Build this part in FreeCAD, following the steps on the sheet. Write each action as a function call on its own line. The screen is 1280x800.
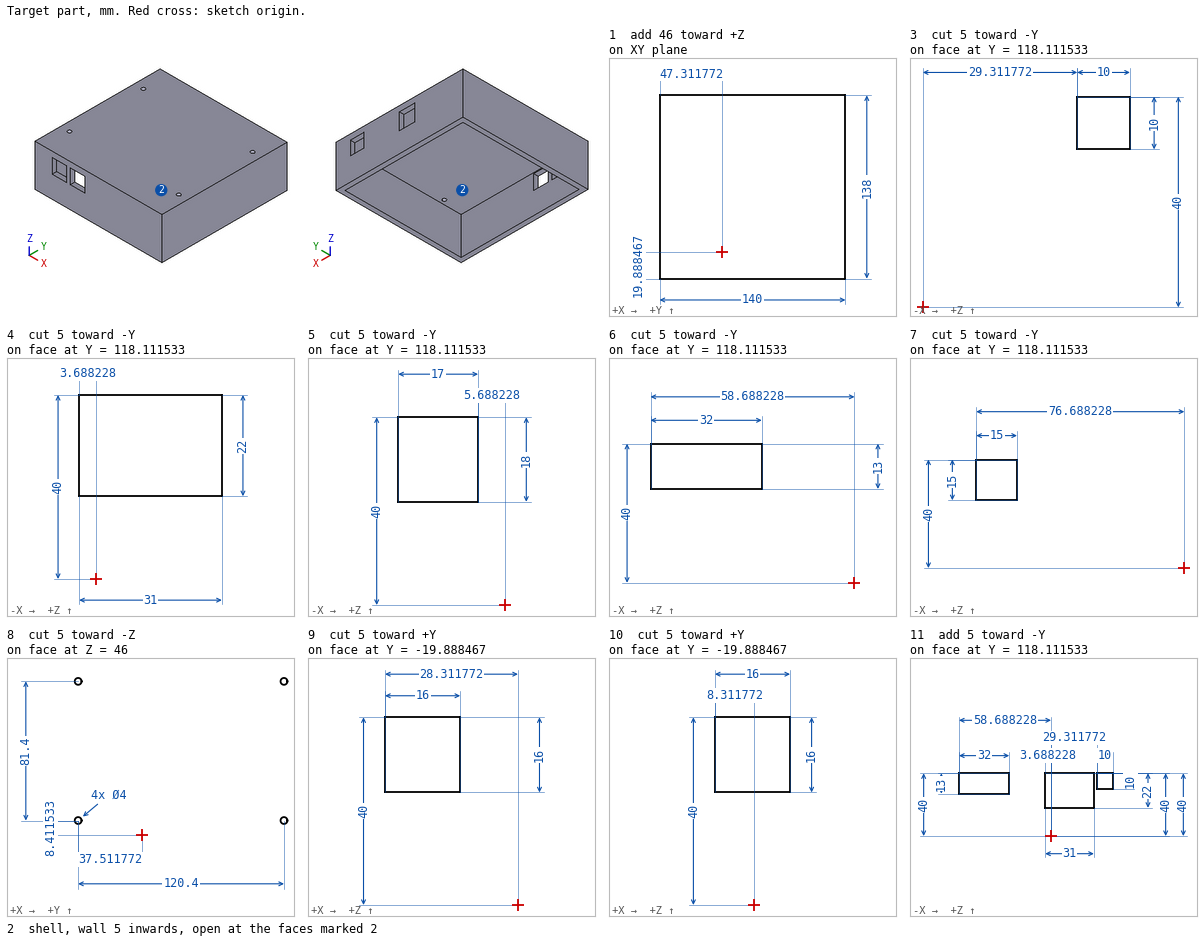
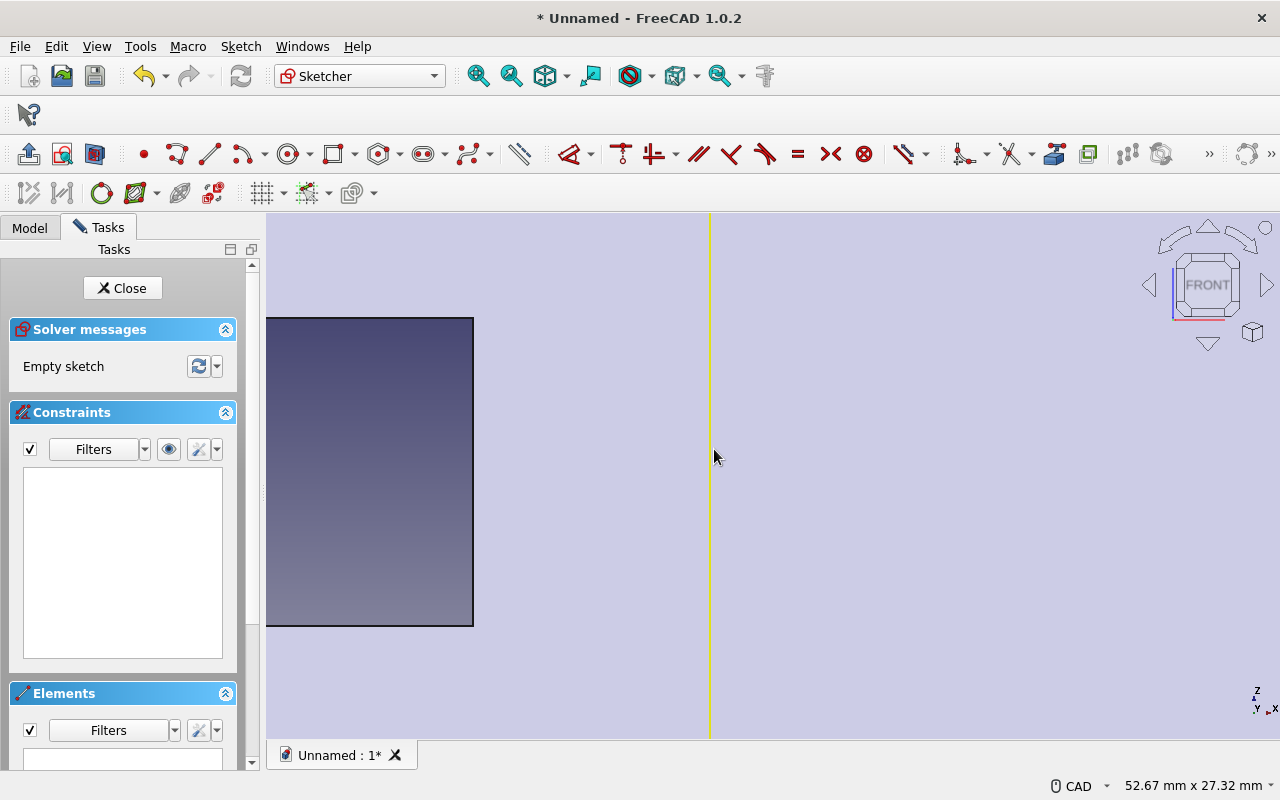
key(g)
key(r)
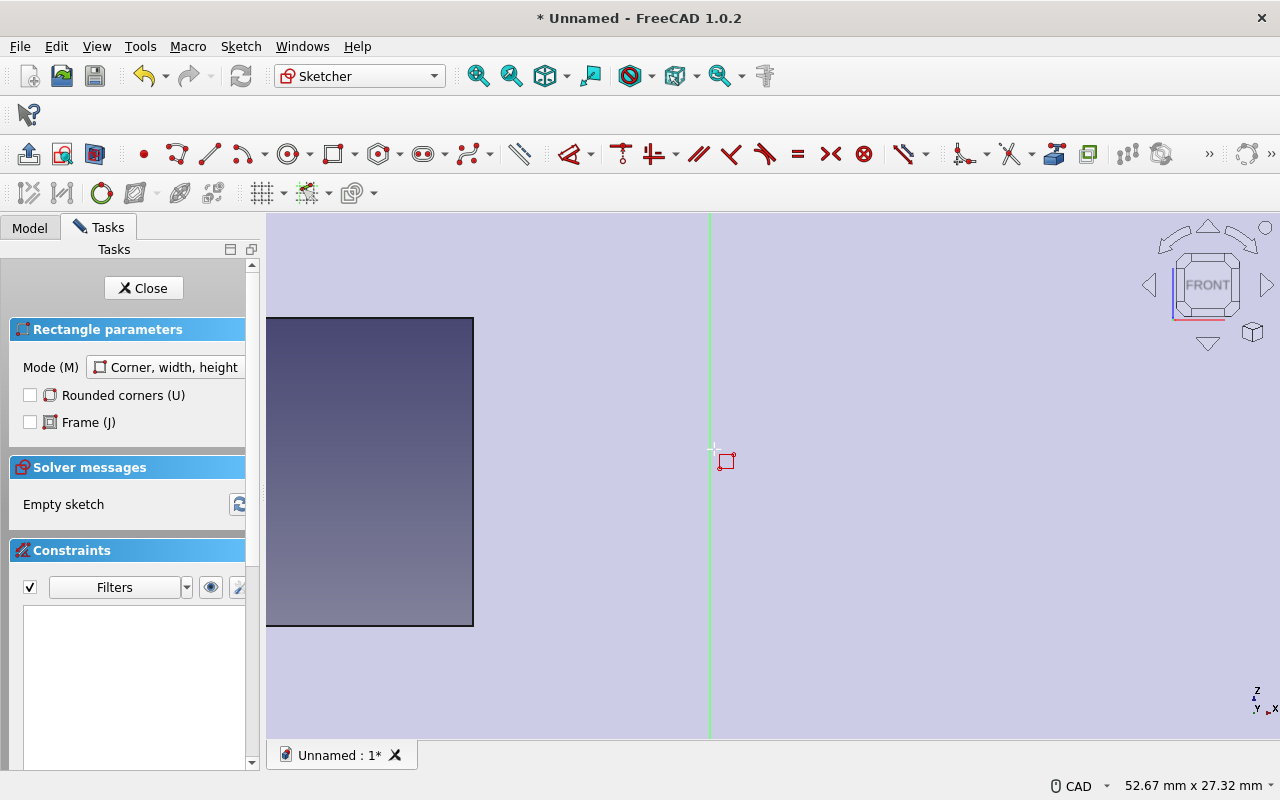
click(550, 318)
move(858, 626)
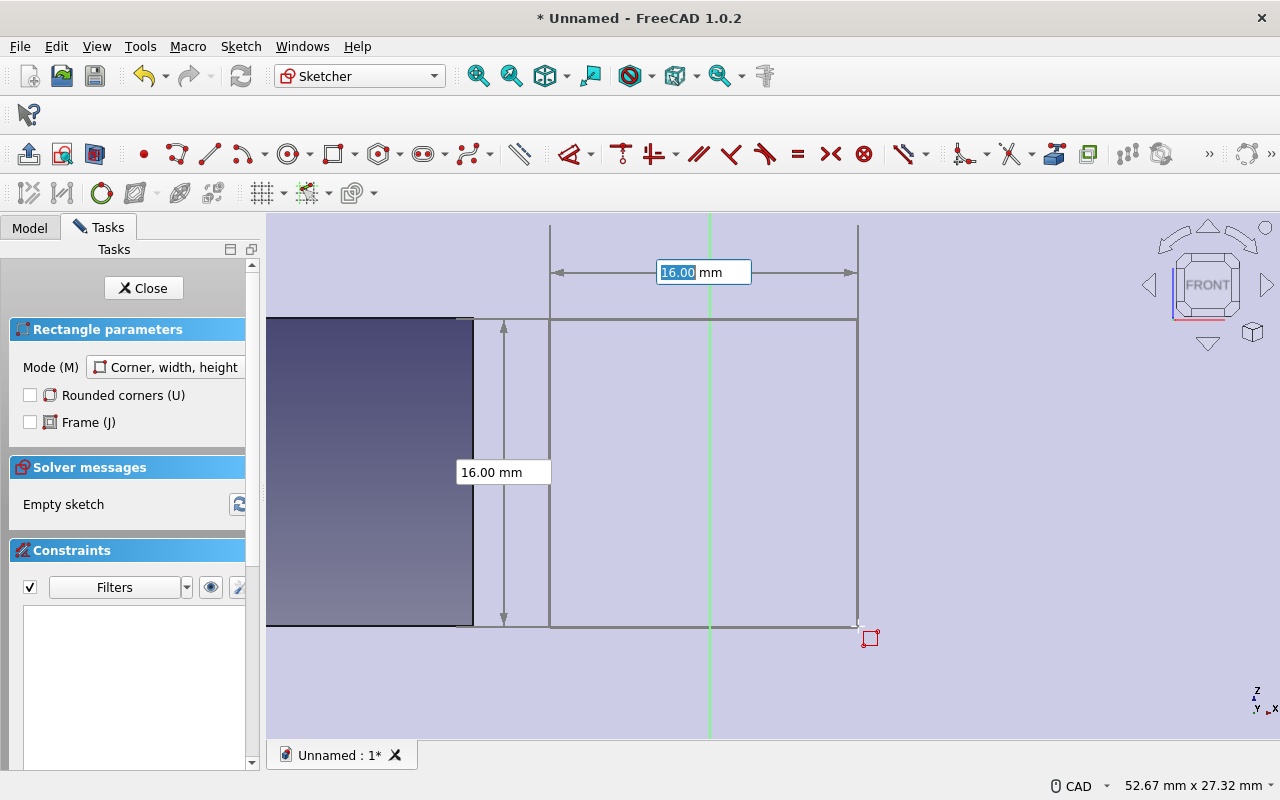
text(16)
key(Tab)
text(16)
key(Return)
key(Escape)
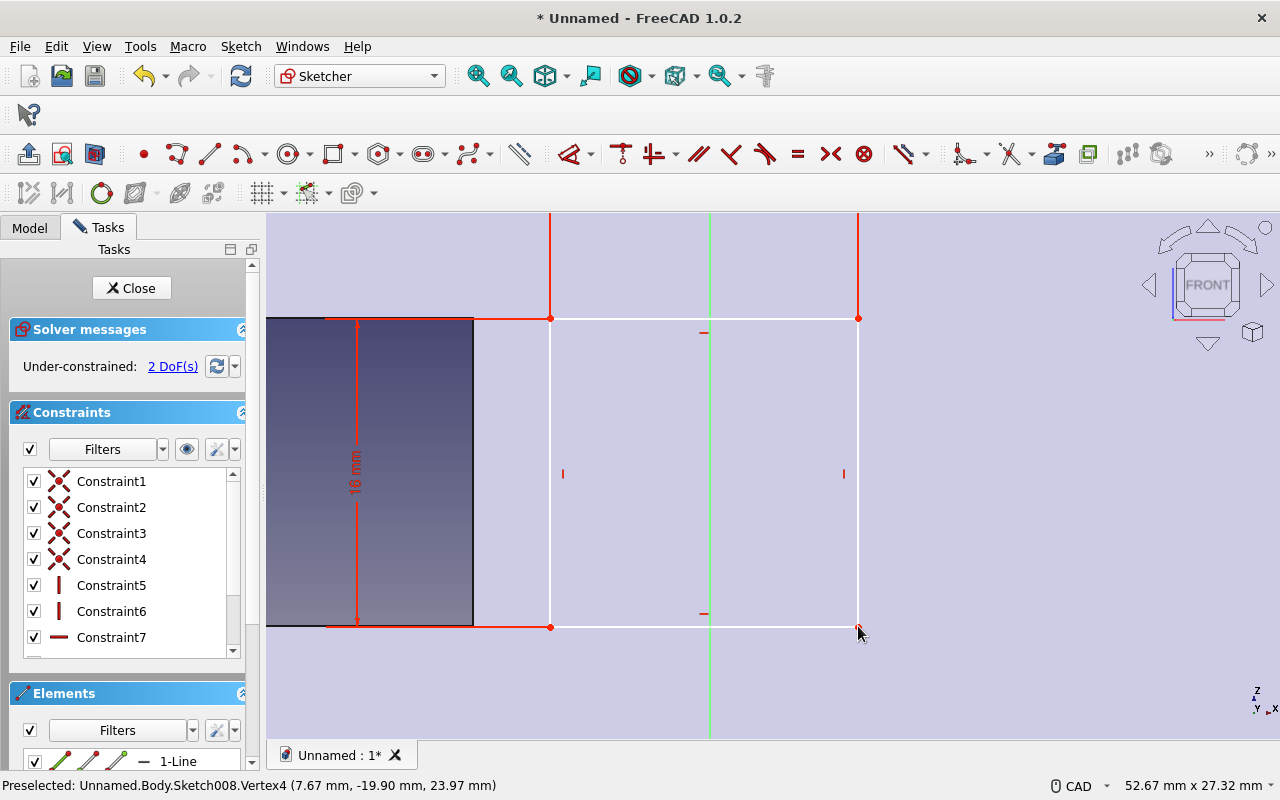
key(d)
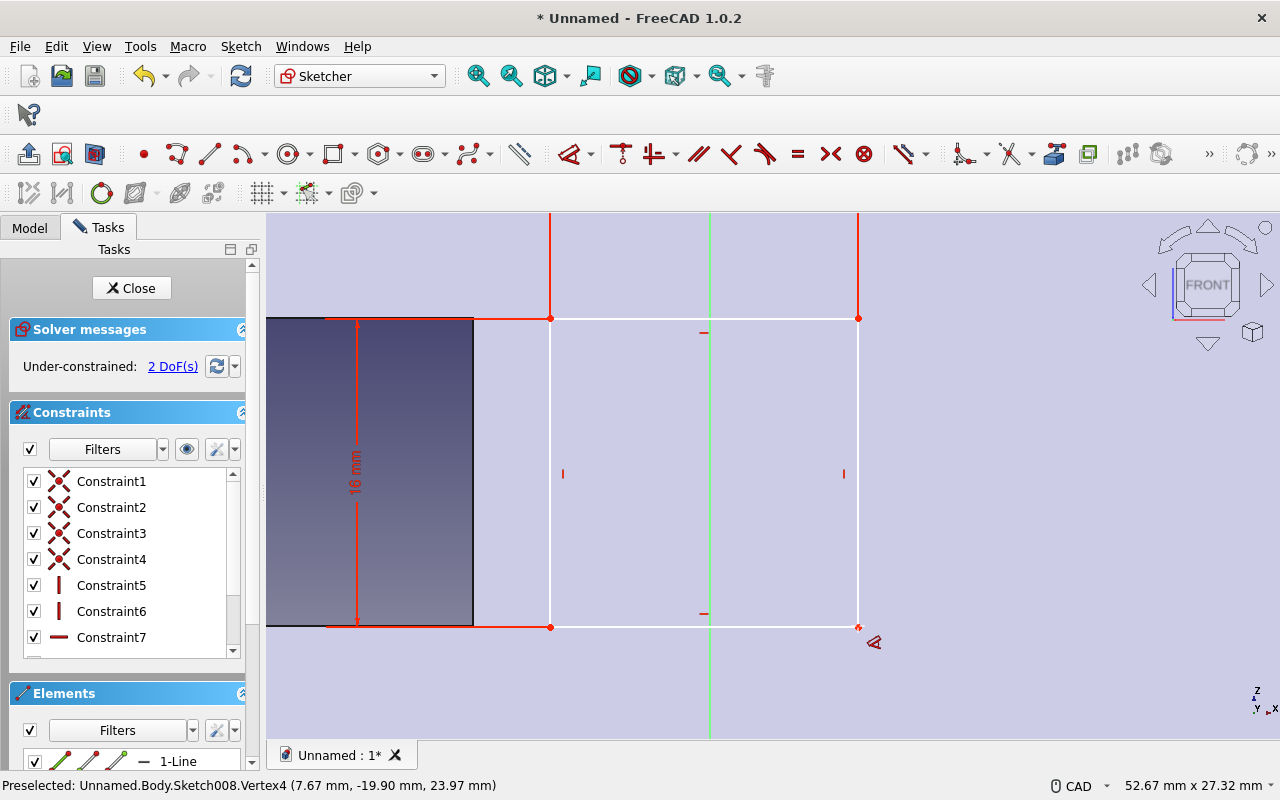
click(550, 319)
click(516, 515)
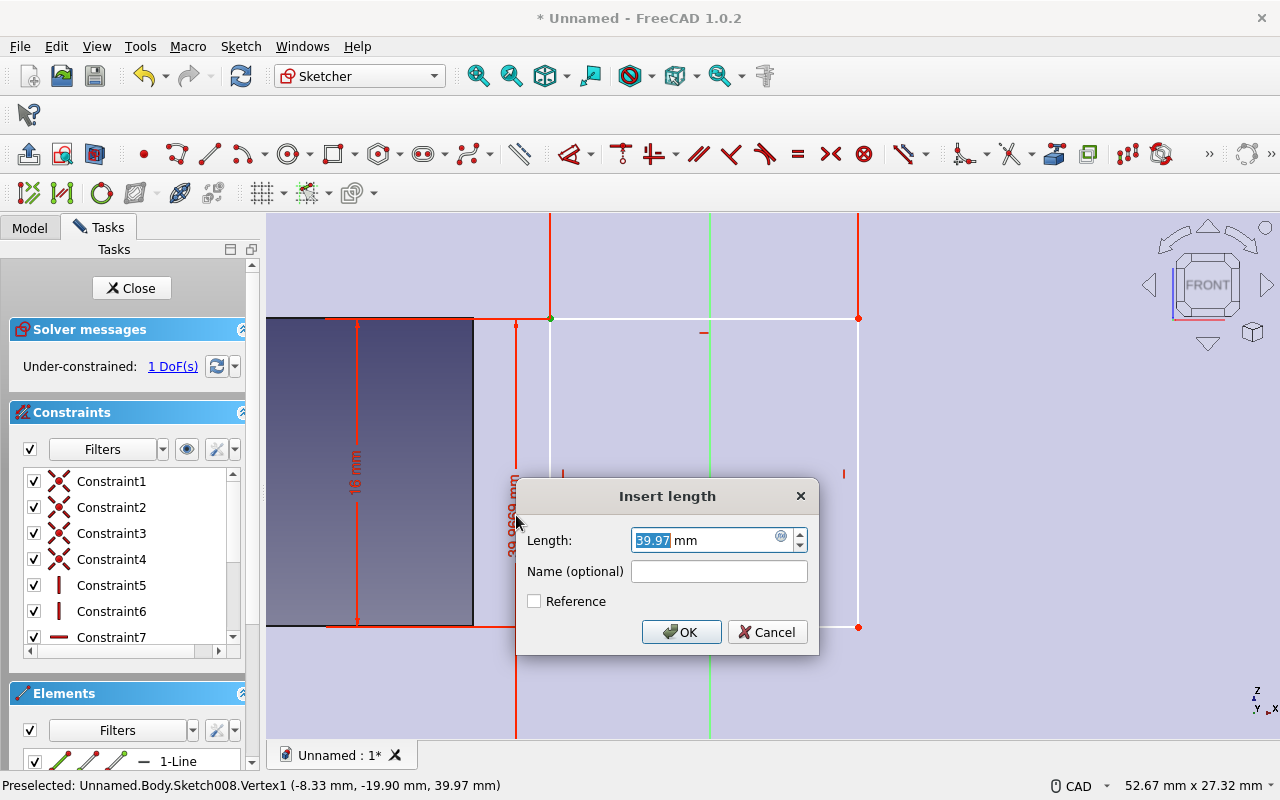
text(40)
key(Return)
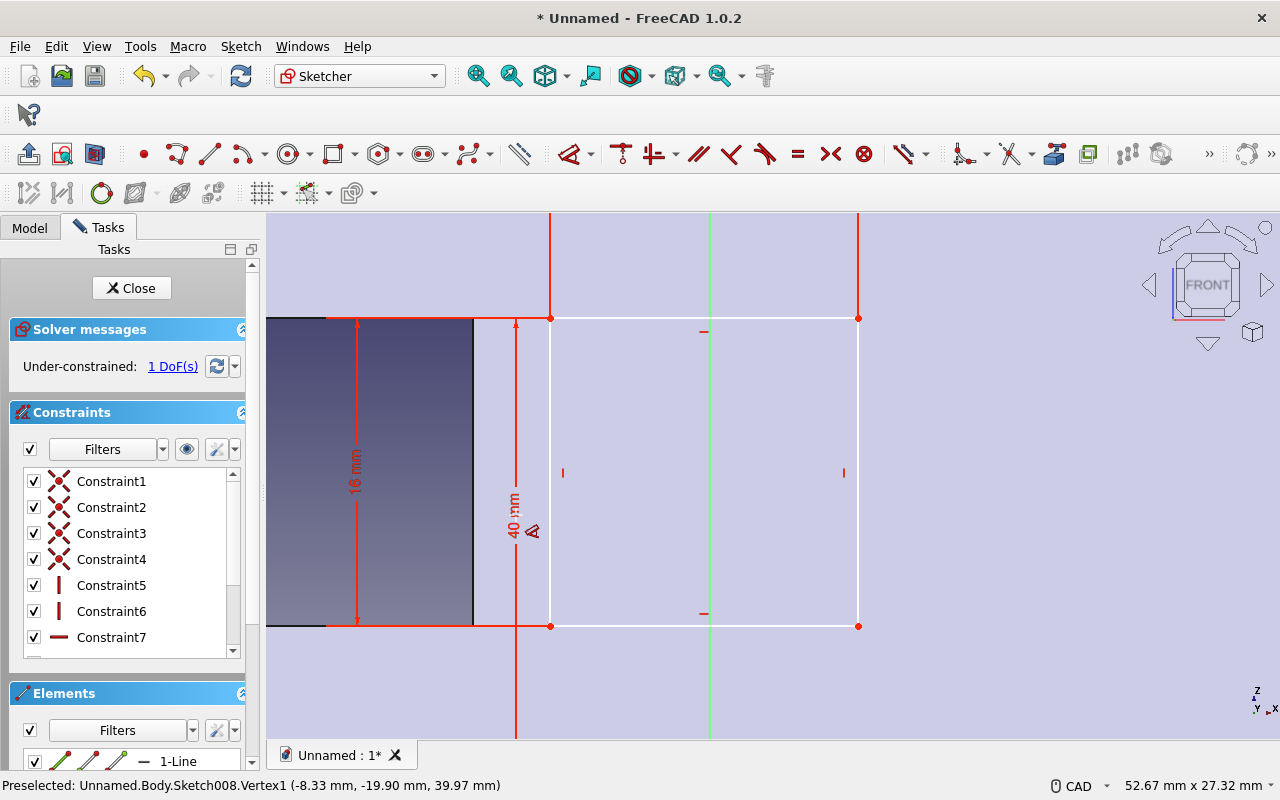
click(550, 318)
click(630, 284)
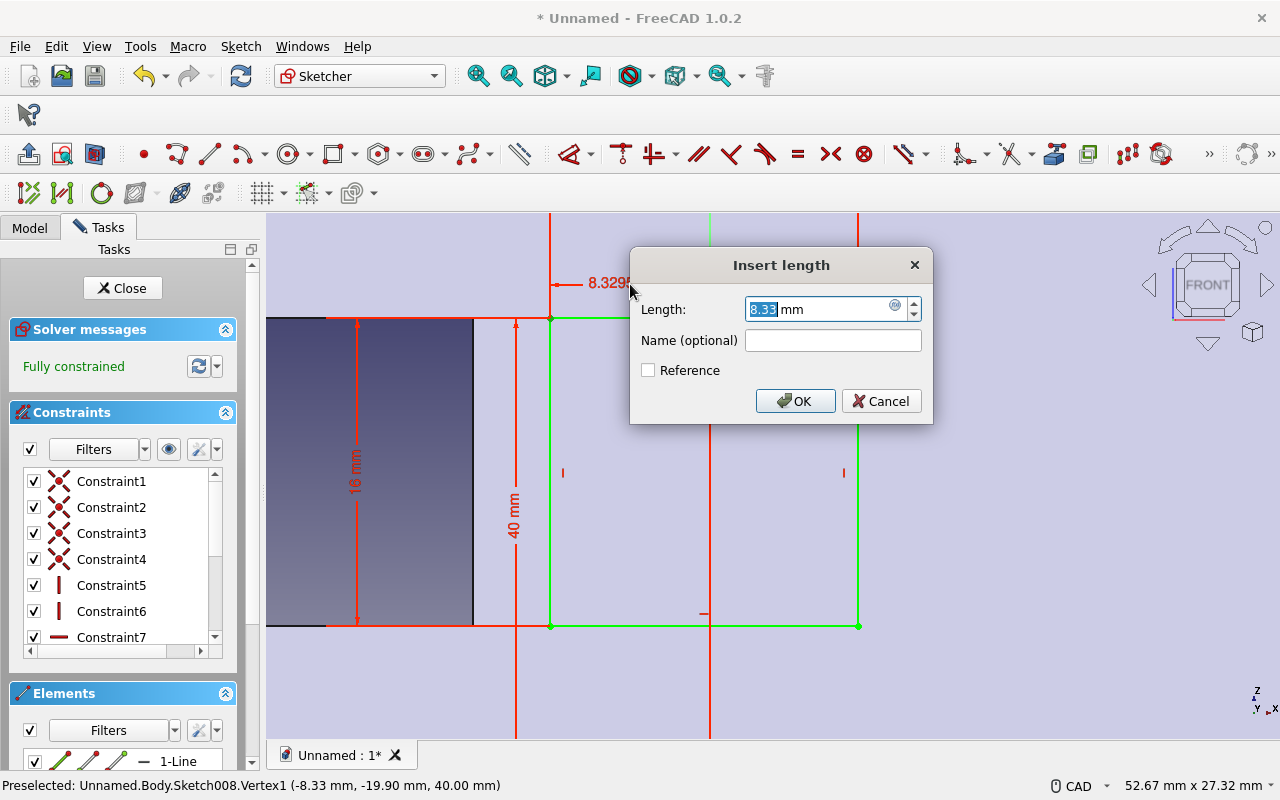
text(8.311772)
key(Return)
key(Escape)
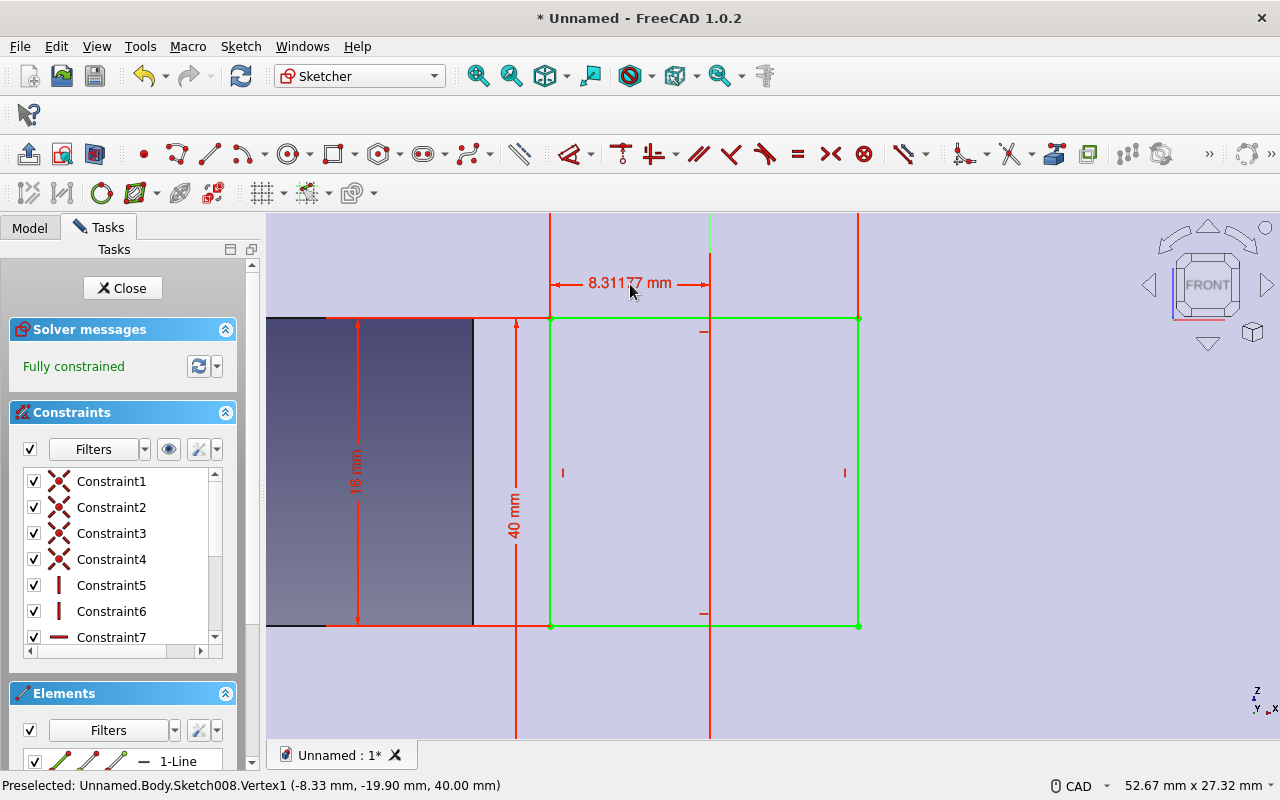
click(123, 288)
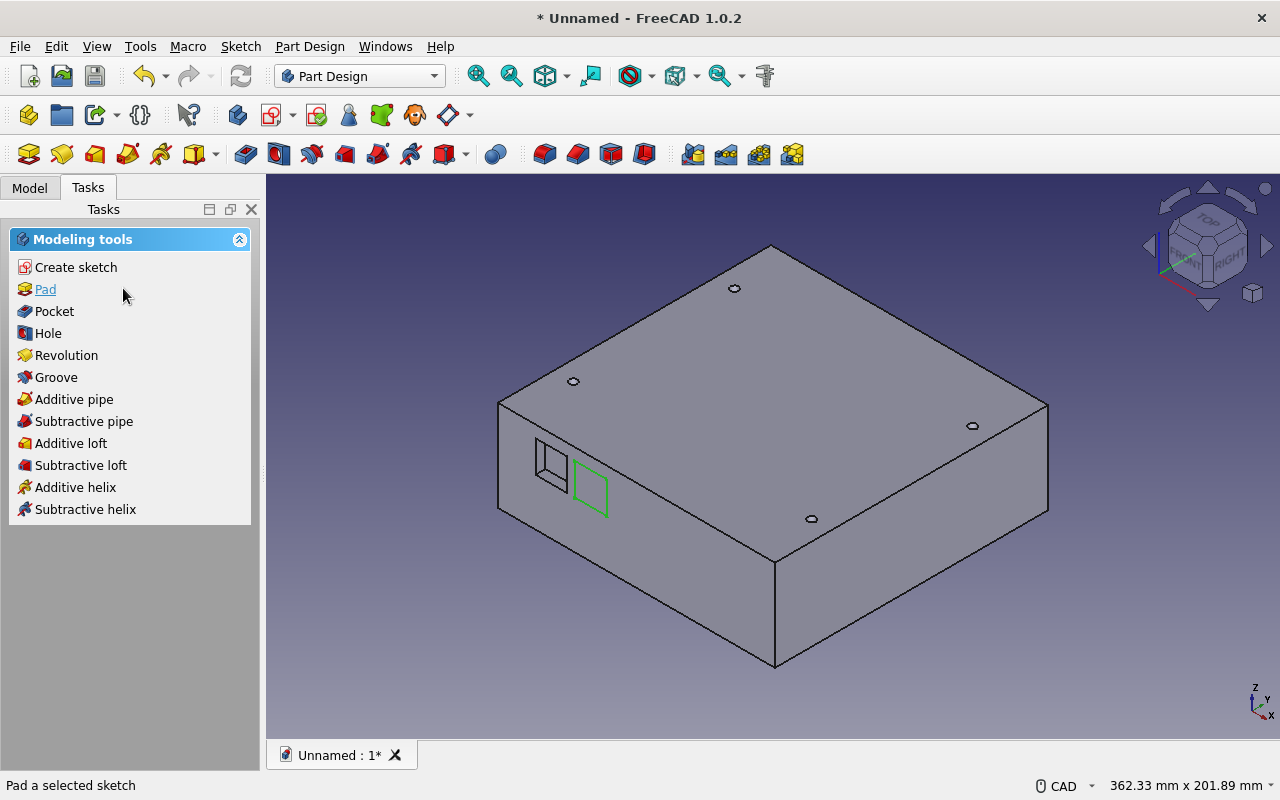
click(246, 154)